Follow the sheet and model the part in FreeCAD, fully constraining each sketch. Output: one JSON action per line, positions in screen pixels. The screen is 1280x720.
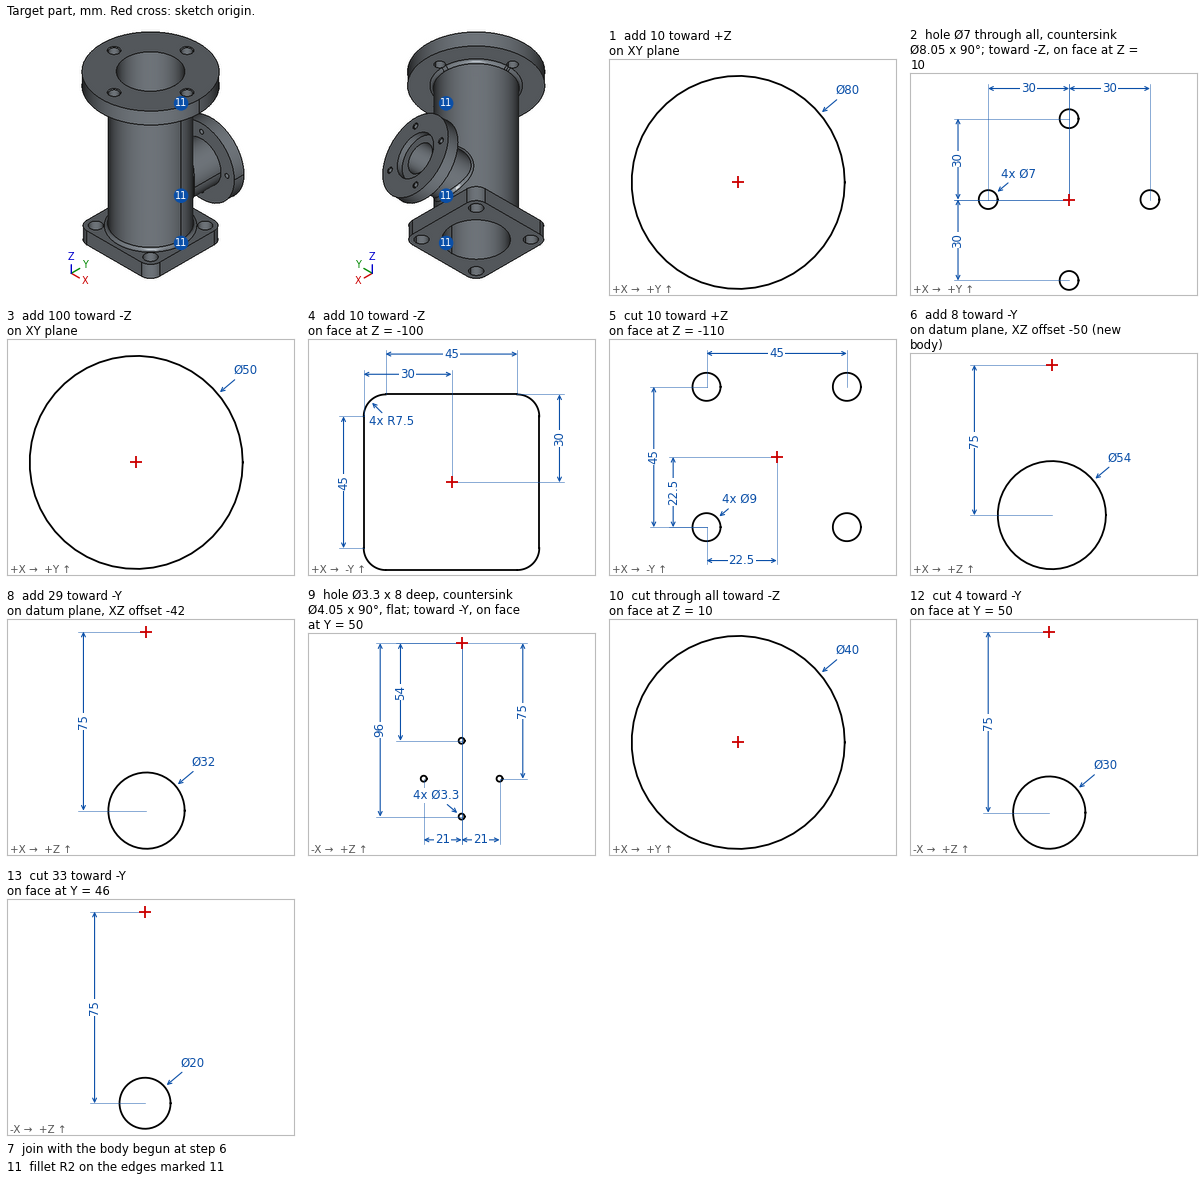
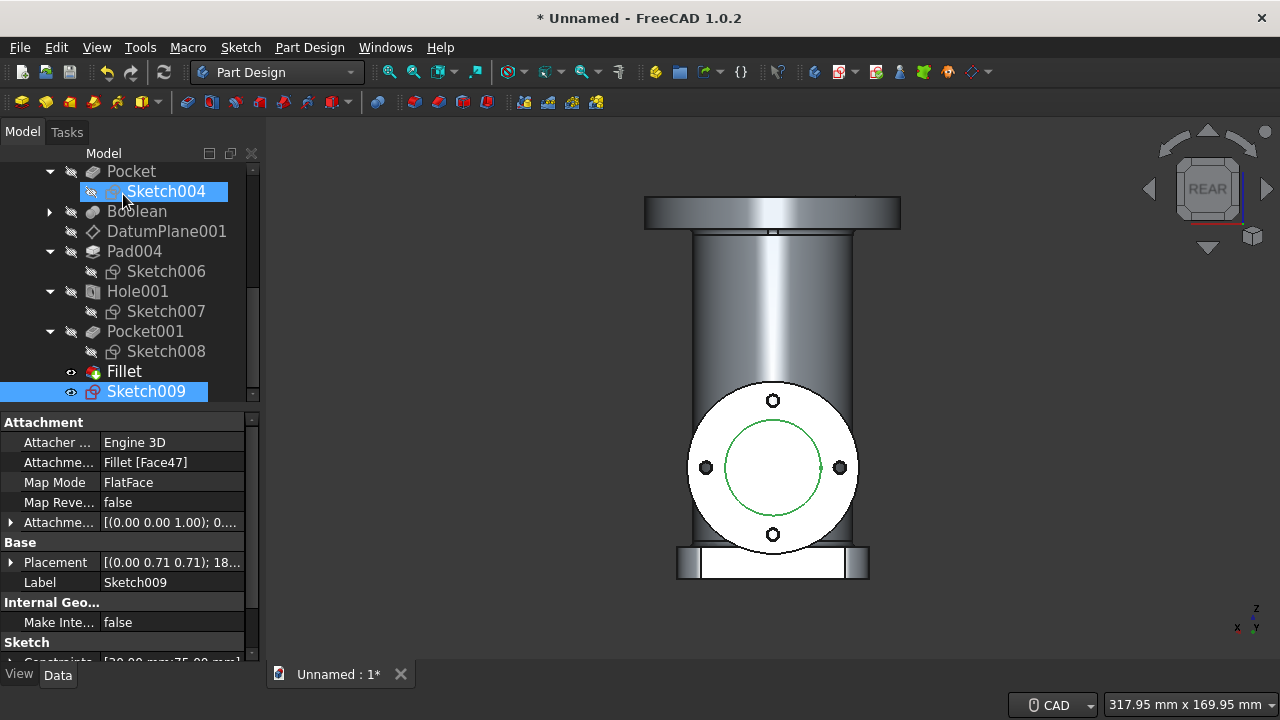
{"action": "left_click", "coordinate": [188, 102]}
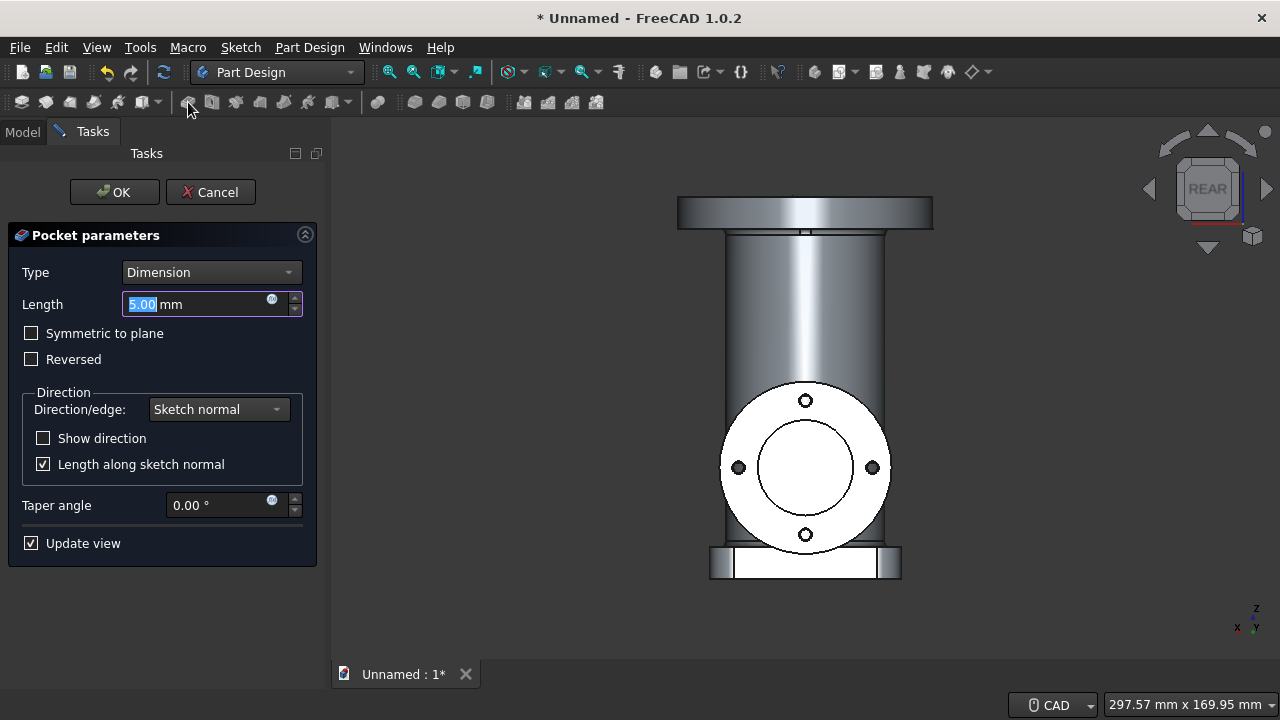
{"action": "type", "text": "4"}
{"action": "key", "text": "Tab"}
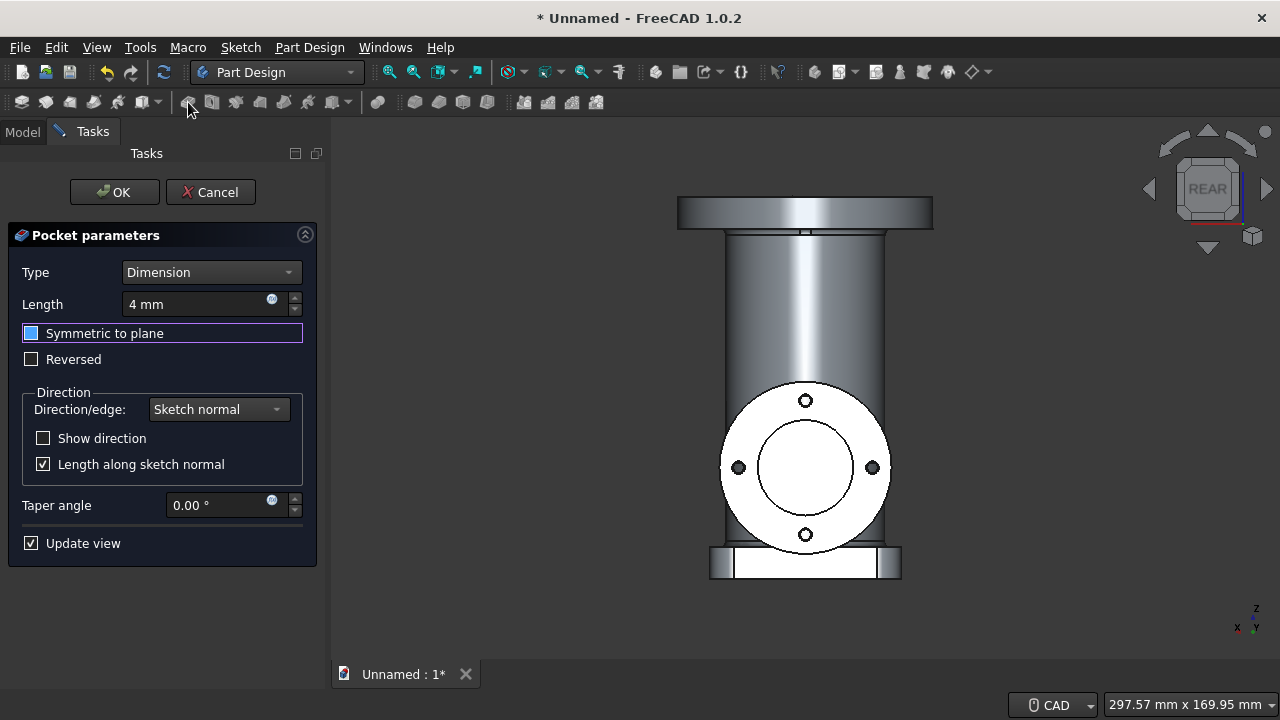
{"action": "left_click", "coordinate": [115, 192]}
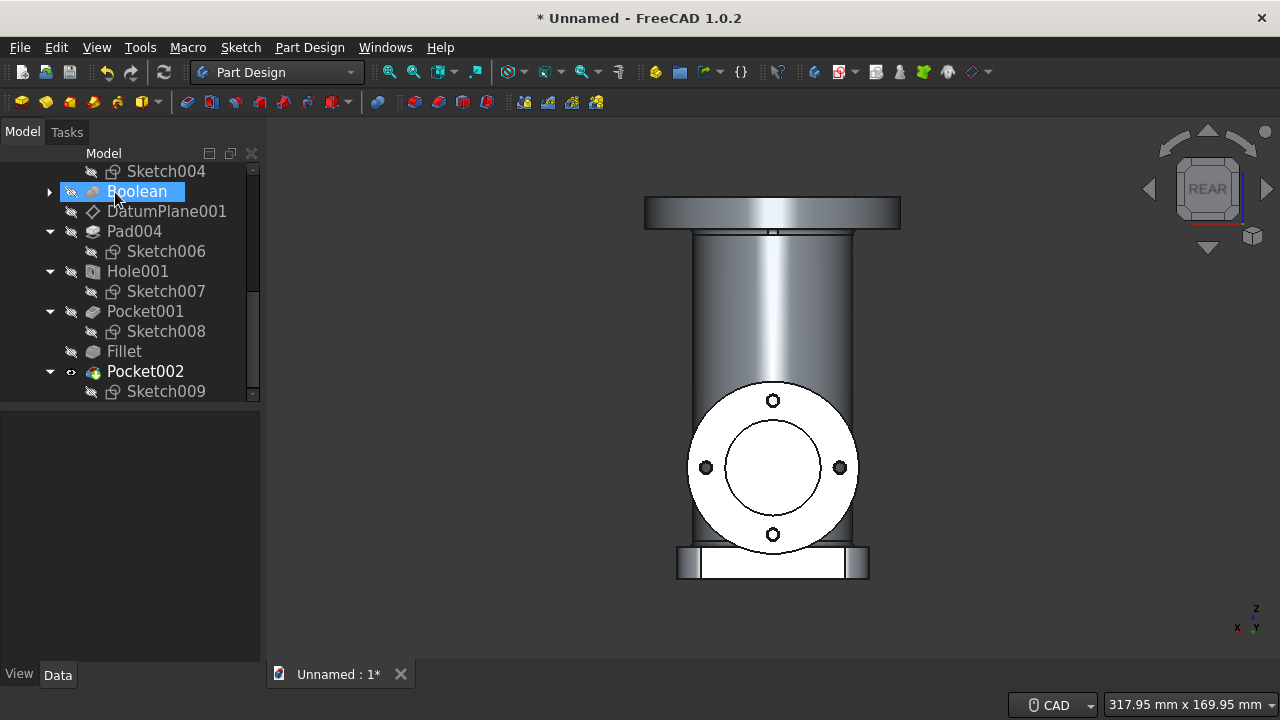
{"action": "left_click", "coordinate": [773, 467]}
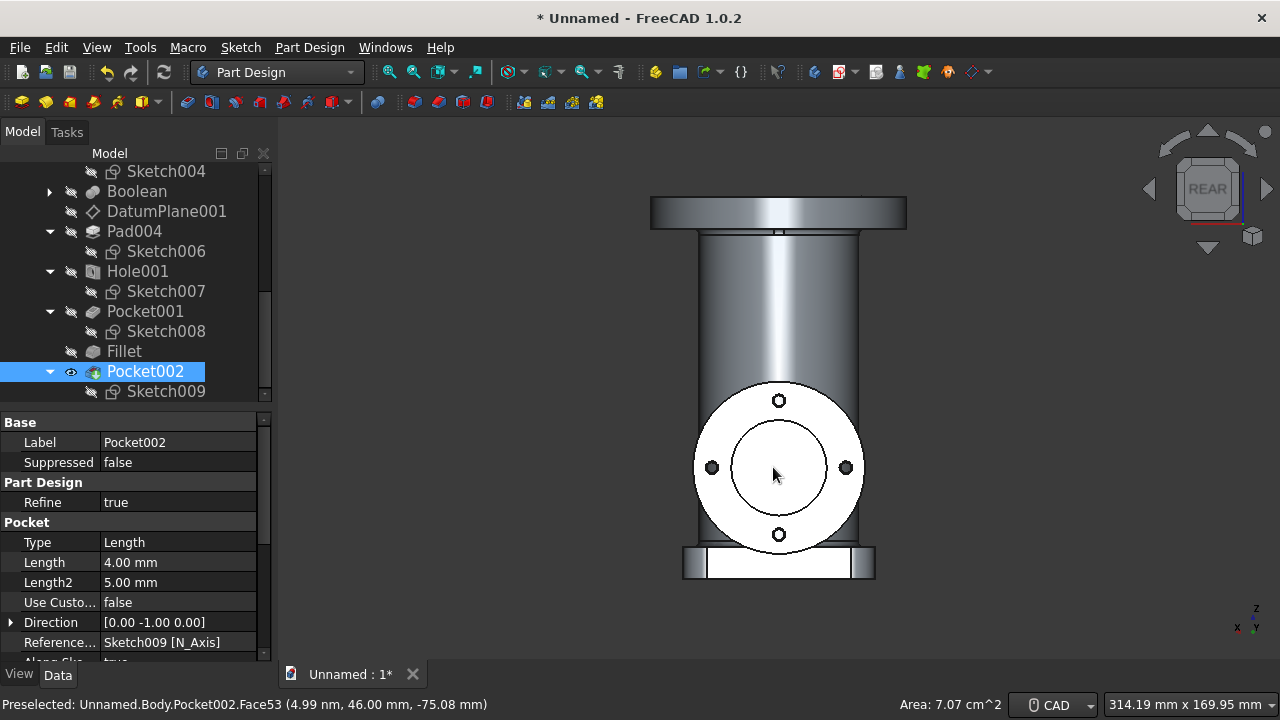
{"action": "left_click", "coordinate": [840, 72]}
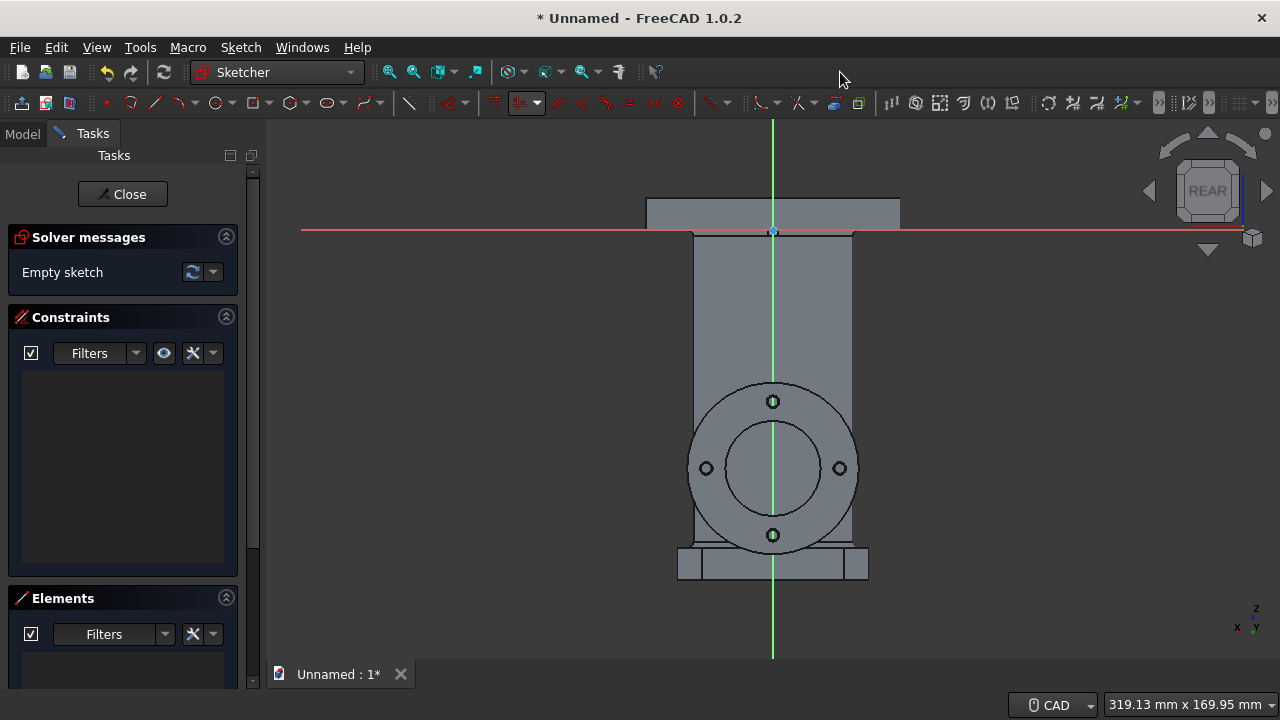
{"action": "left_click", "coordinate": [70, 104]}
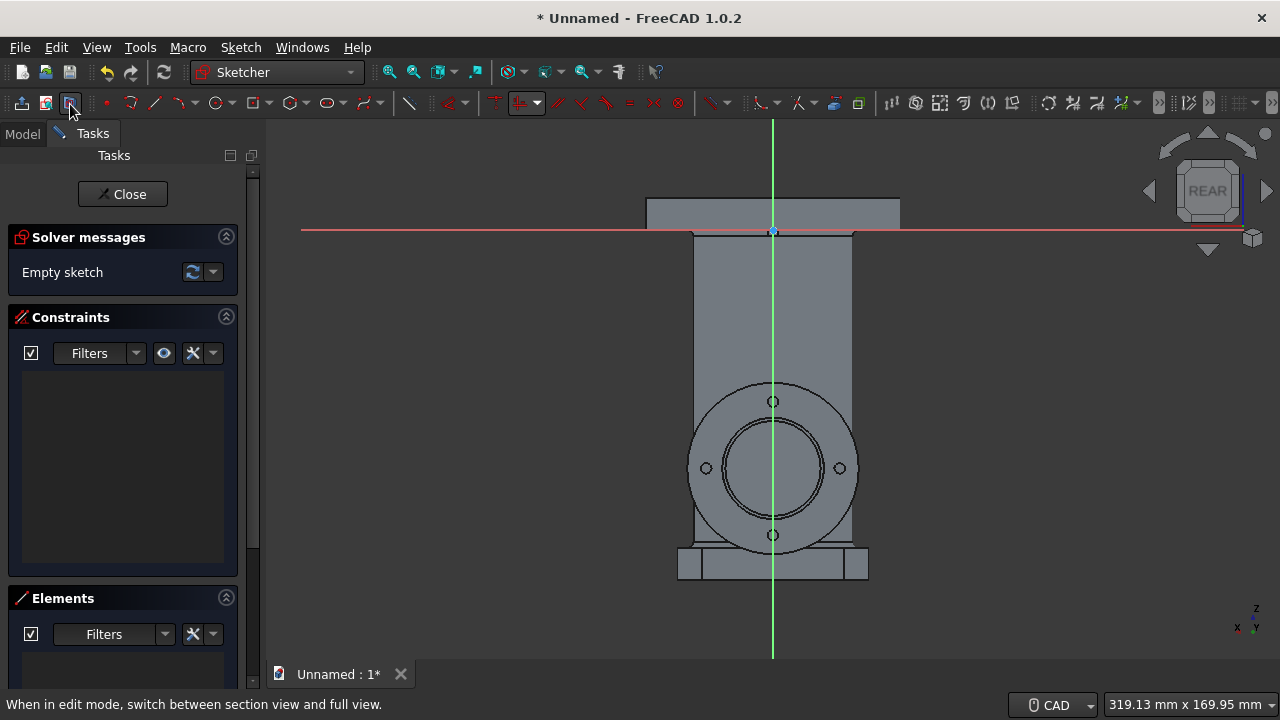
{"action": "scroll", "coordinate": [790, 489], "scroll_direction": "up", "scroll_amount": 8}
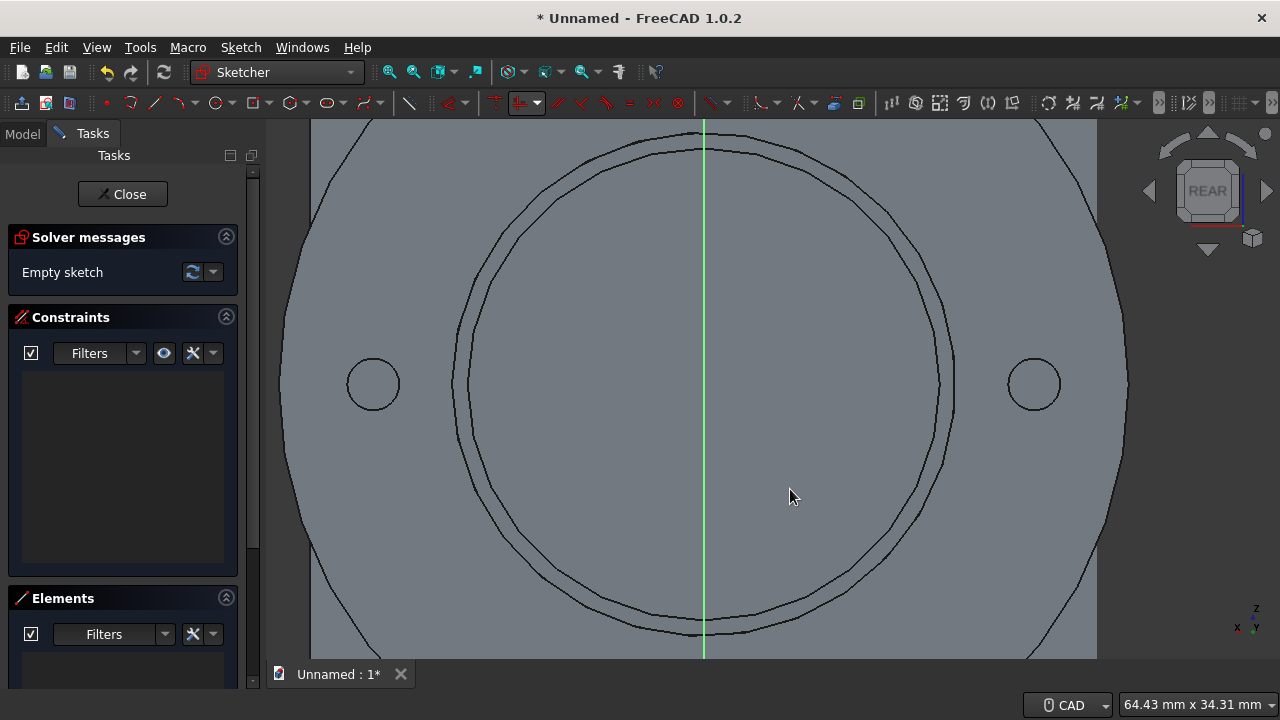
{"action": "left_click", "coordinate": [216, 104]}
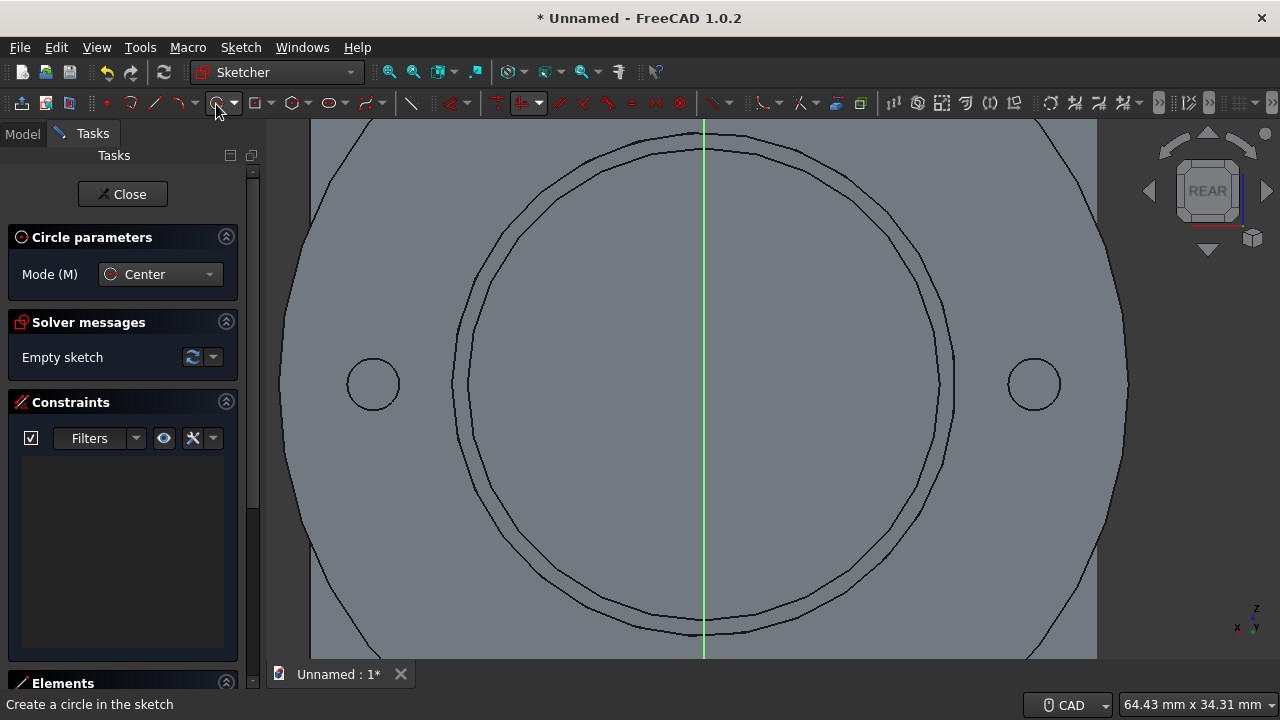
{"action": "left_click", "coordinate": [704, 384]}
{"action": "mouse_move", "coordinate": [815, 273]}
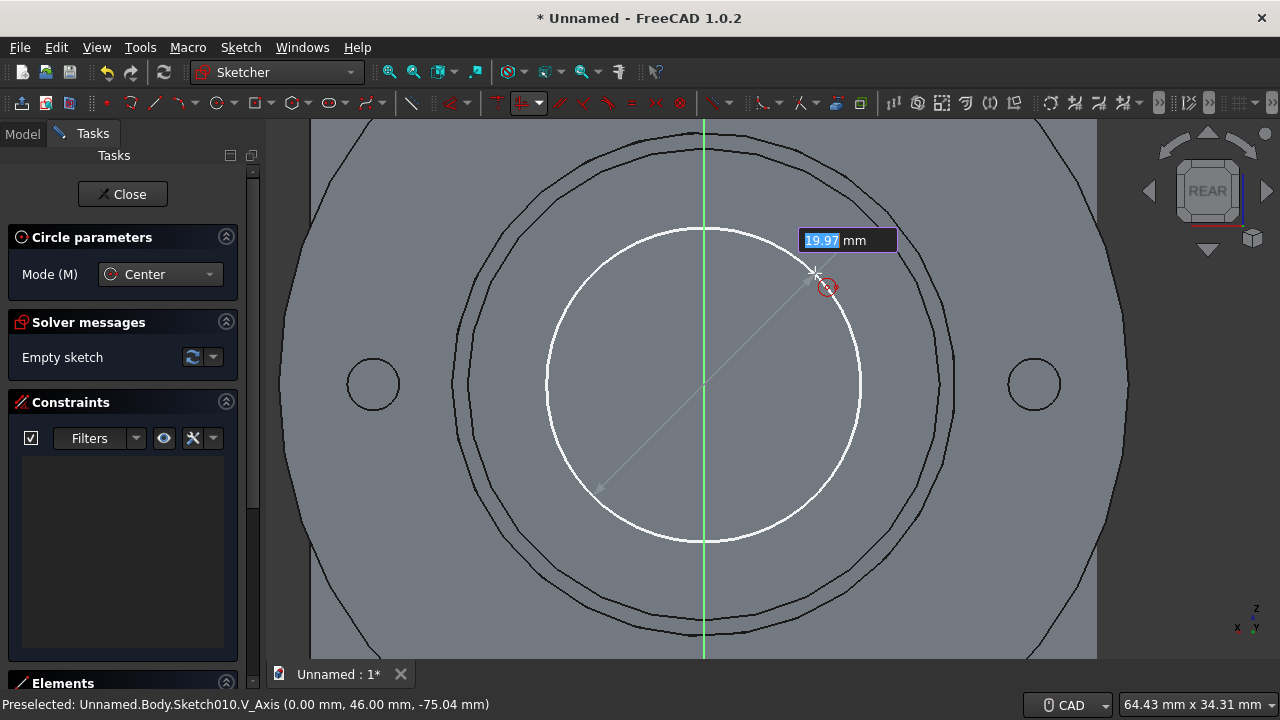
{"action": "type", "text": "20"}
{"action": "key", "text": "Return"}
{"action": "key", "text": "Escape"}